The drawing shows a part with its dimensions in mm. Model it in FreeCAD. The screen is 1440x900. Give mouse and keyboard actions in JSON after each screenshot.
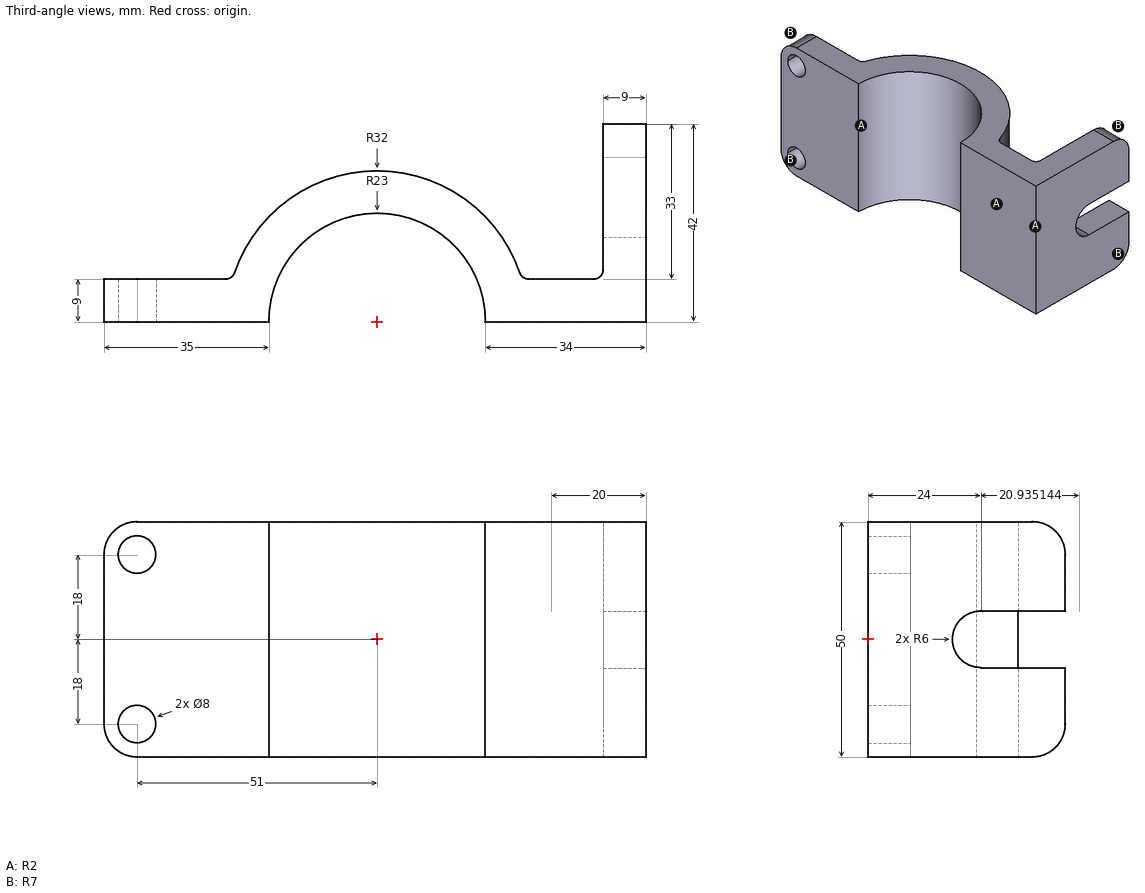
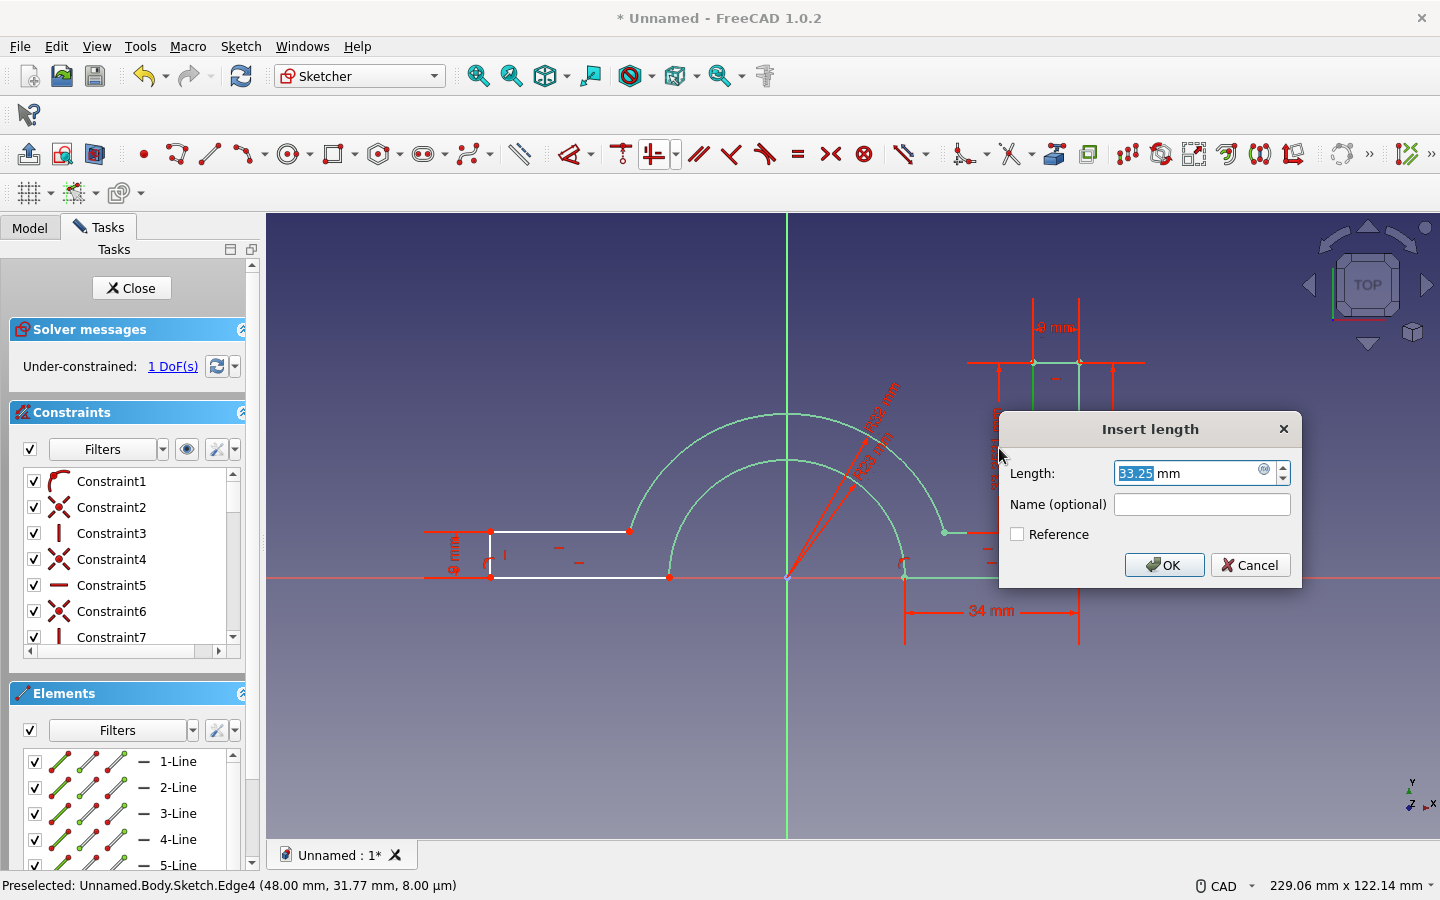
{"action": "type", "text": "33"}
{"action": "key", "text": "Return"}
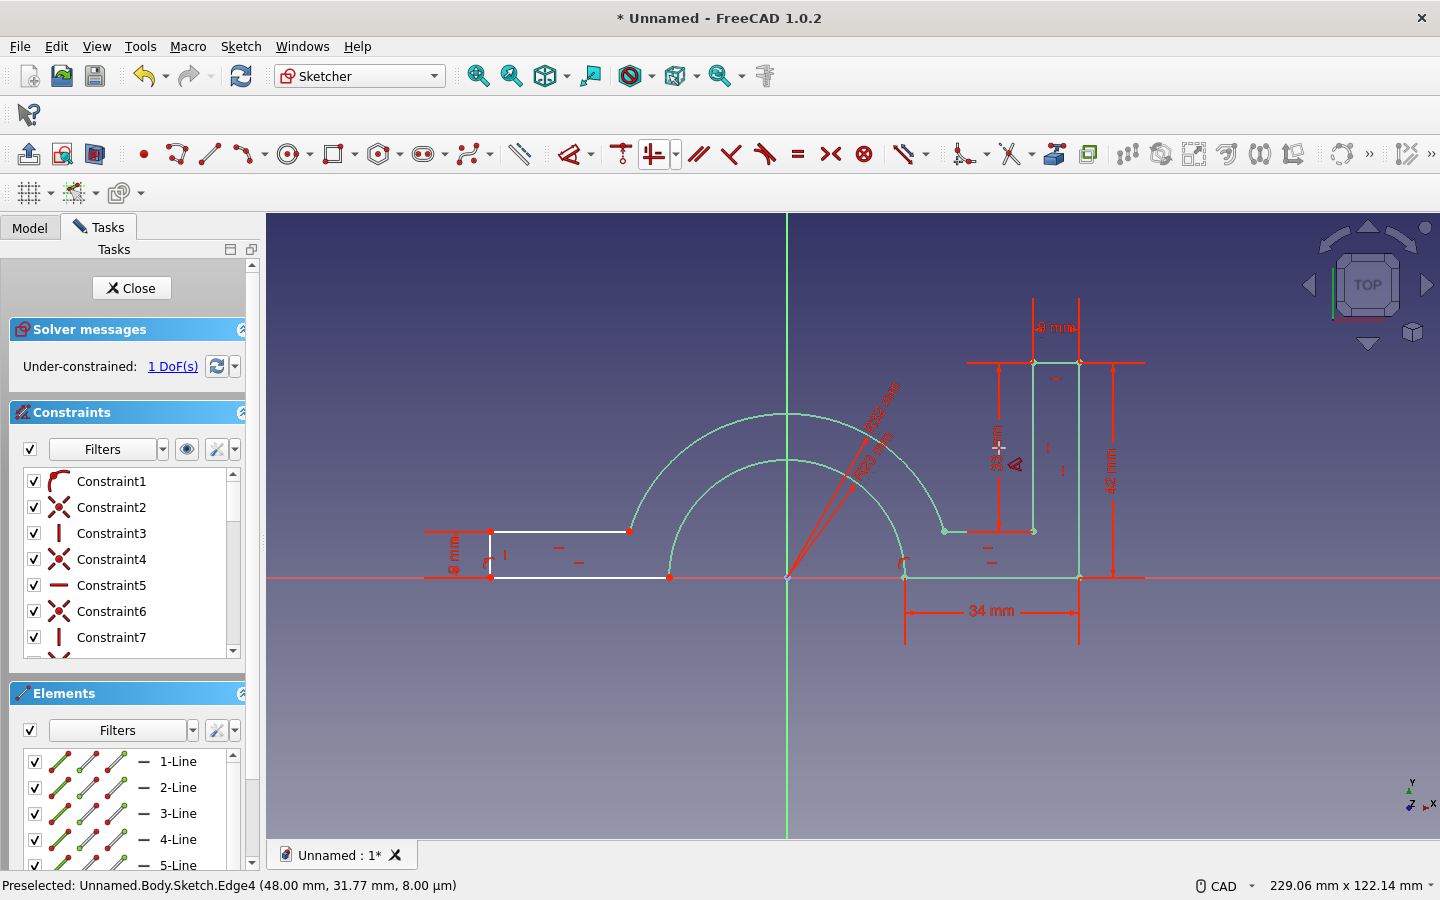
{"action": "left_click", "coordinate": [544, 578]}
{"action": "left_click", "coordinate": [580, 612]}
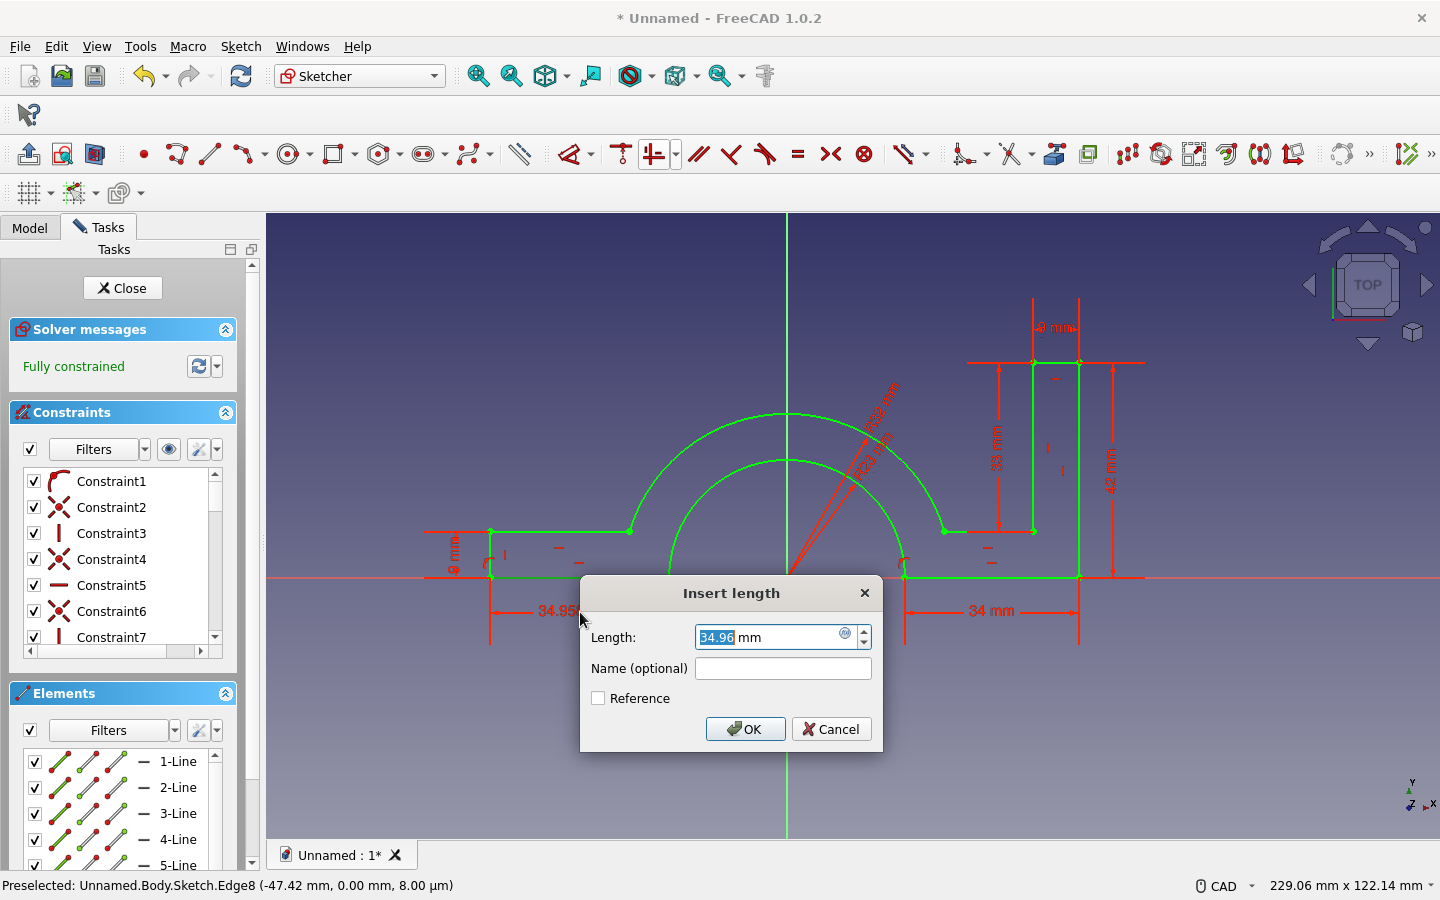
{"action": "type", "text": "35"}
{"action": "key", "text": "Return"}
{"action": "key", "text": "Escape"}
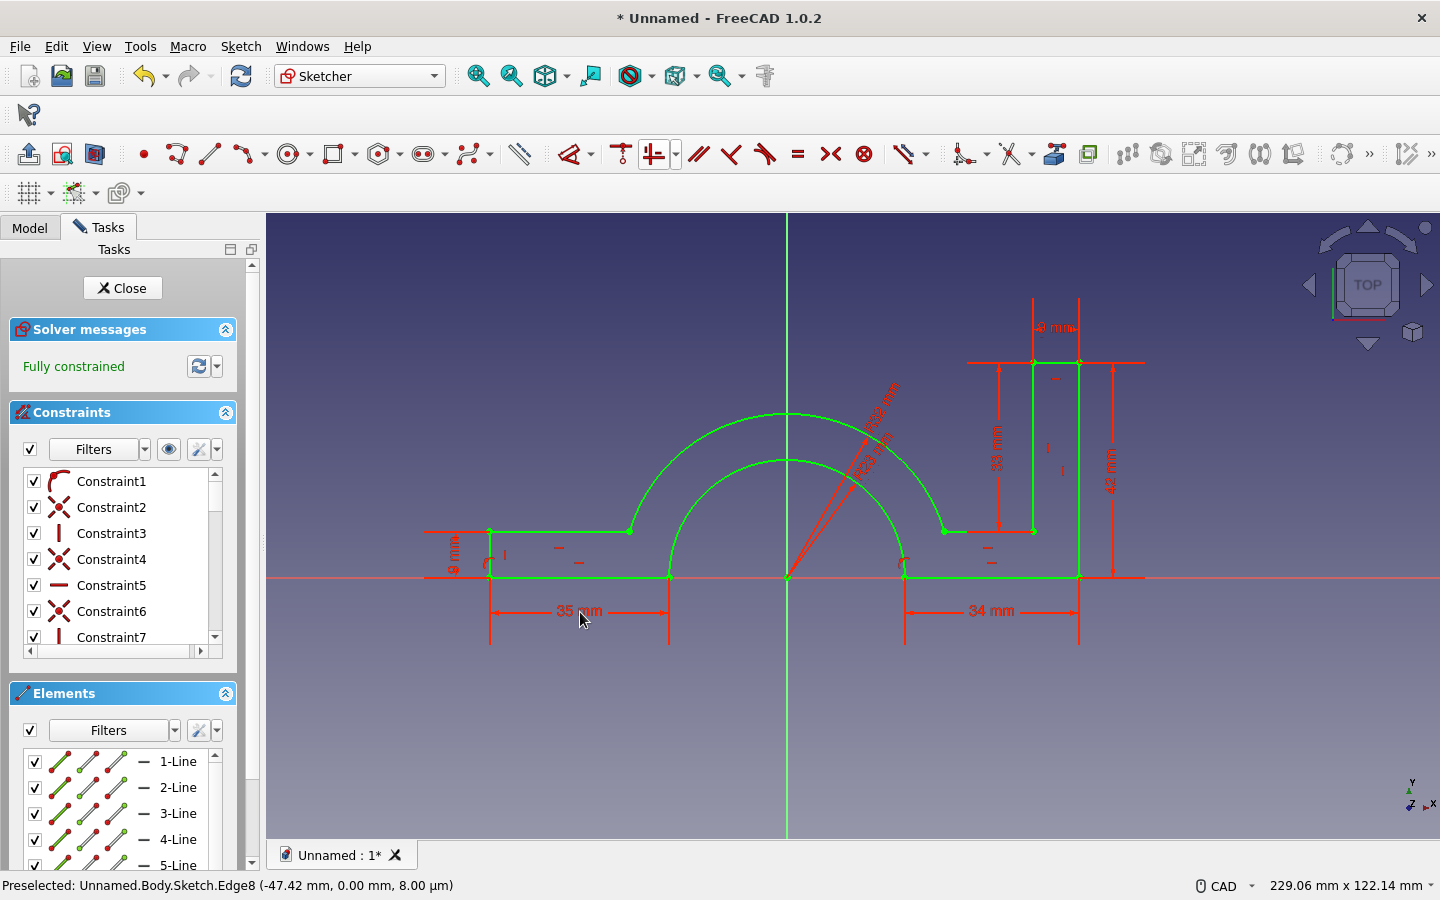
{"action": "left_click", "coordinate": [123, 288]}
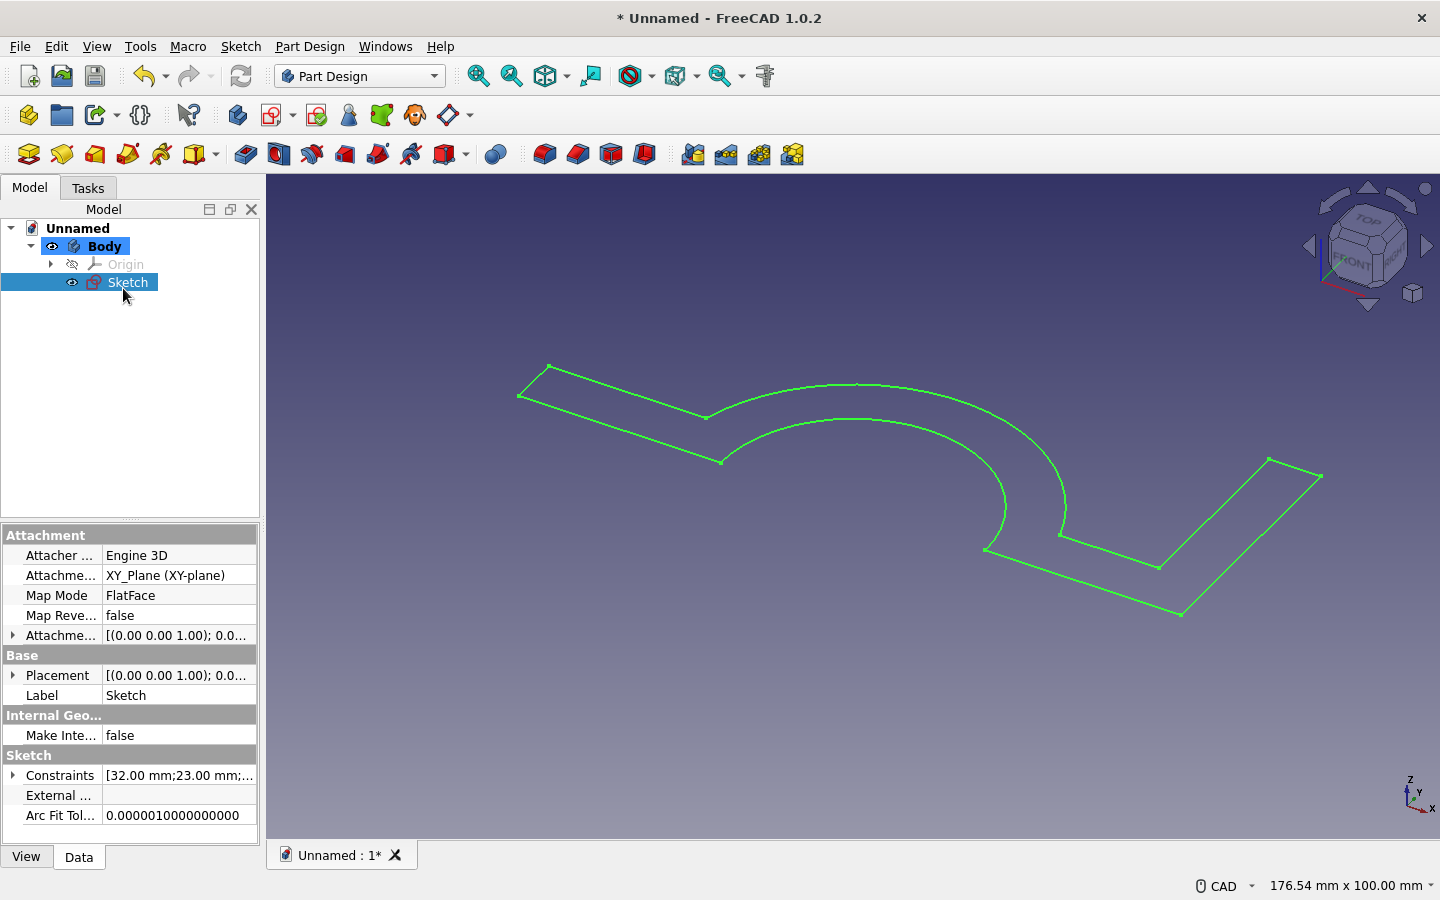
{"action": "left_click", "coordinate": [29, 154]}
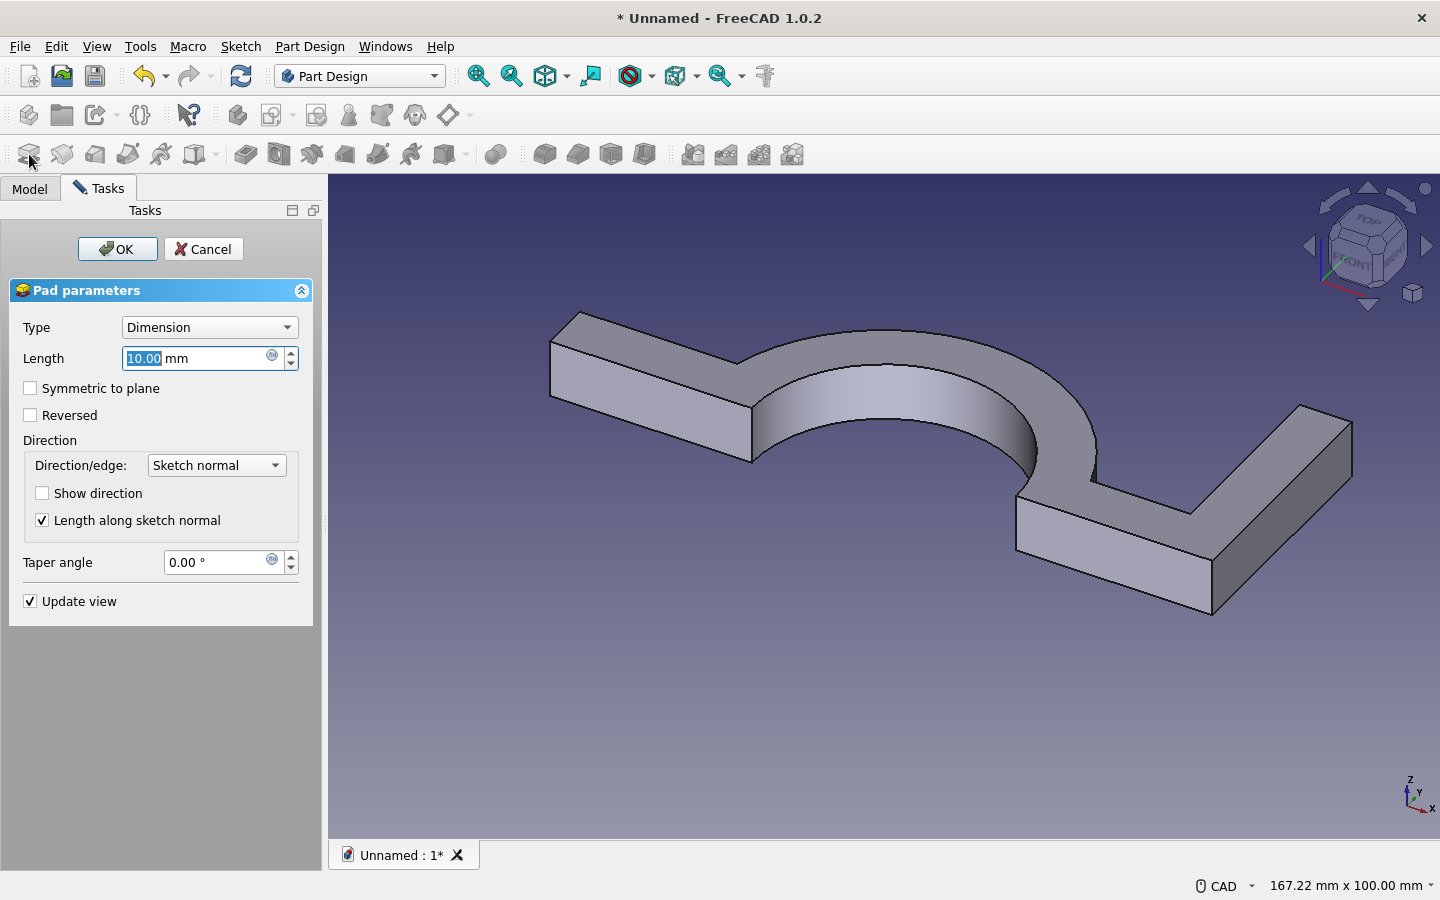
{"action": "type", "text": "50"}
{"action": "key", "text": "Tab"}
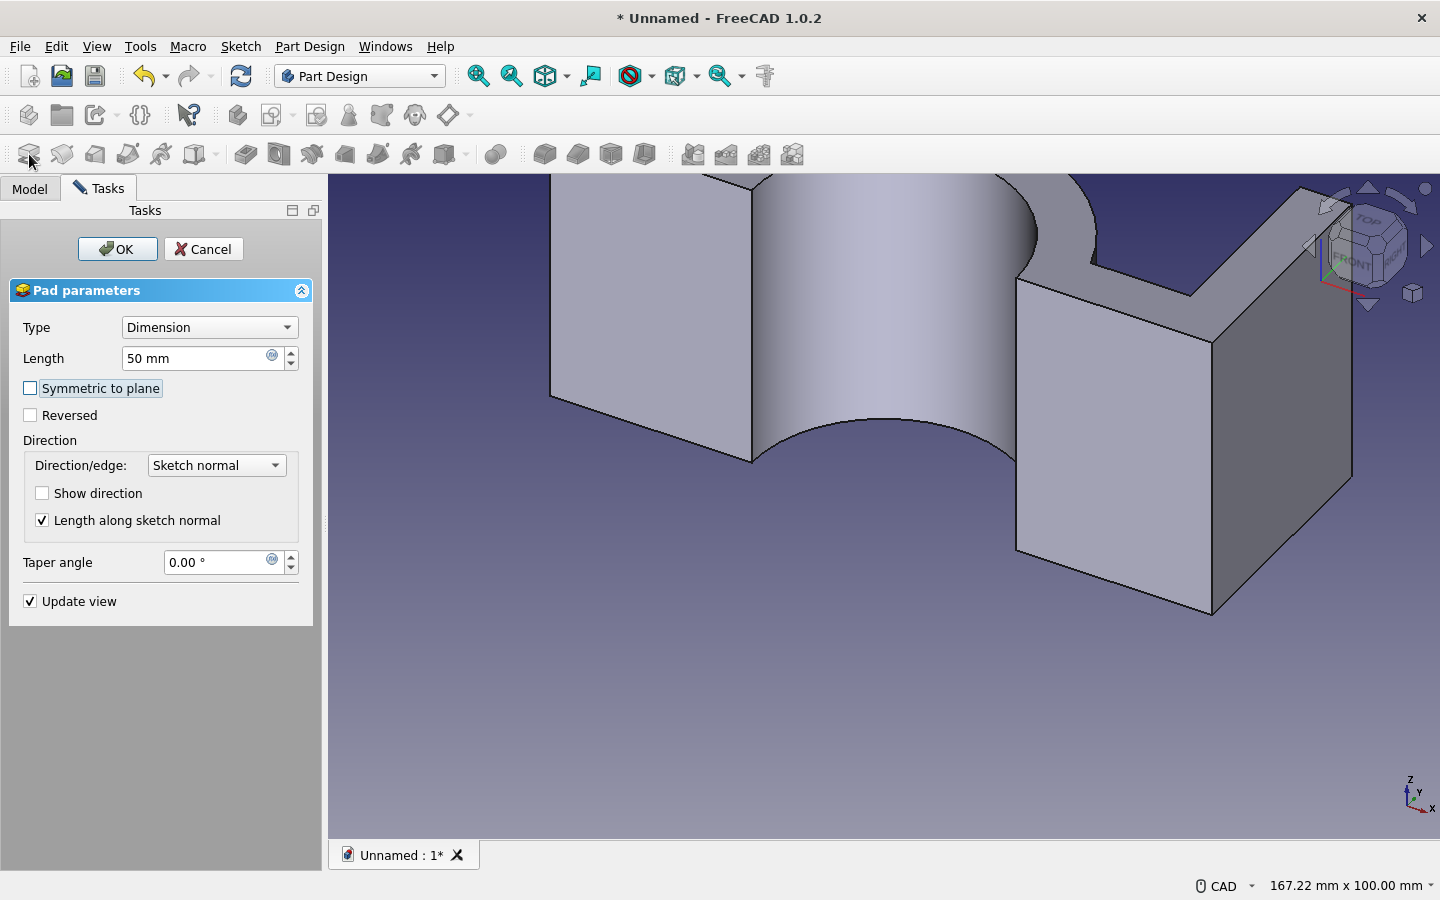
{"action": "left_click", "coordinate": [31, 388]}